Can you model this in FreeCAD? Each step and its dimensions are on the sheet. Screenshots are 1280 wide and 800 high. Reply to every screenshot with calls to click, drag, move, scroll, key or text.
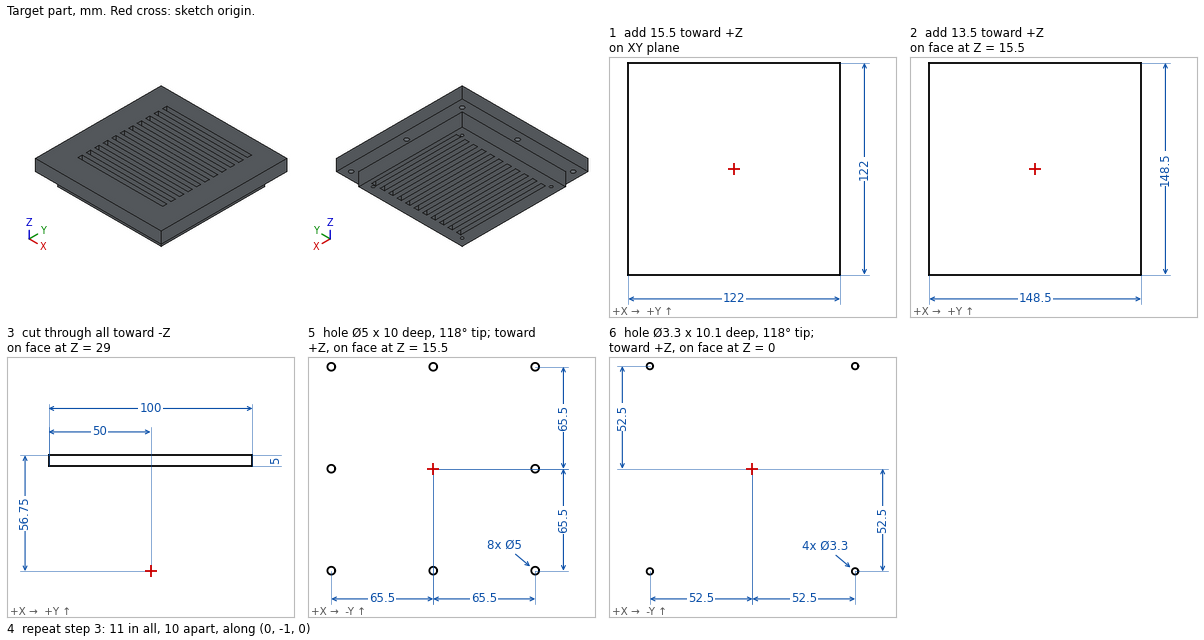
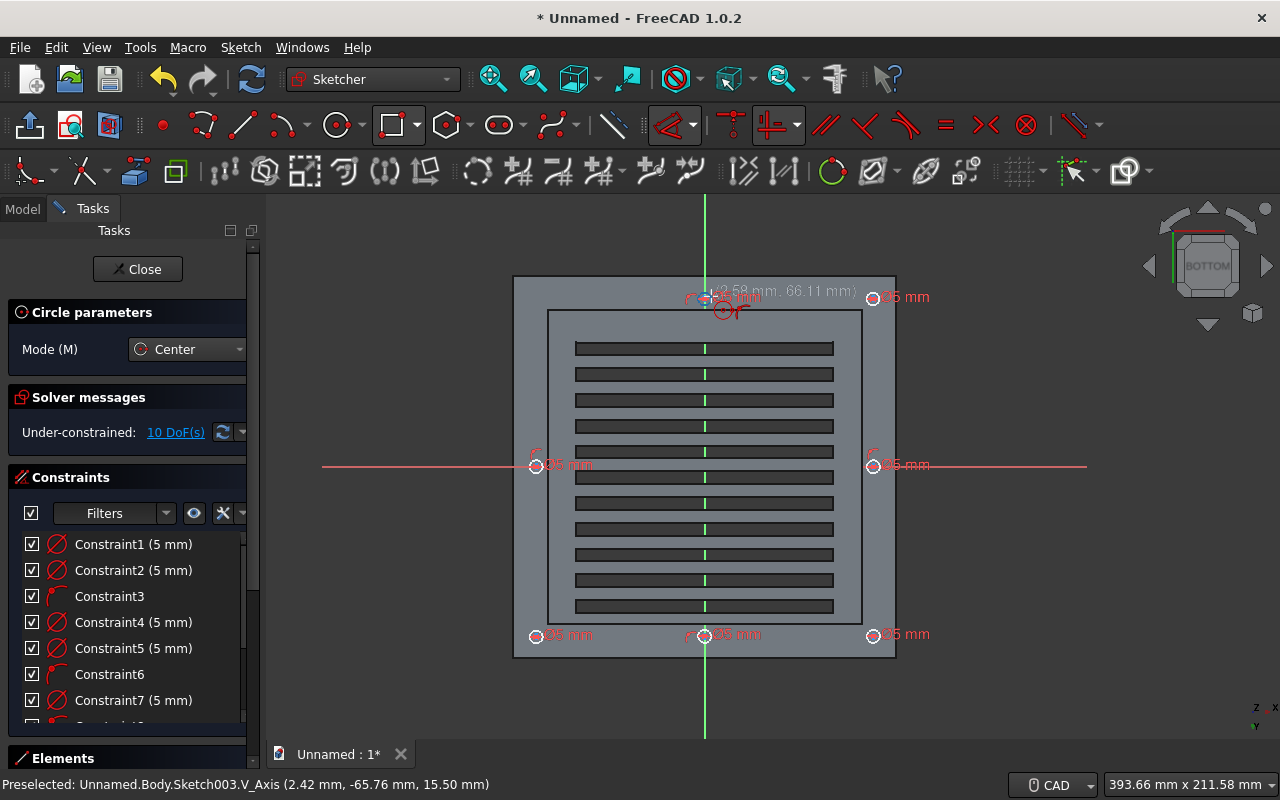
scroll(536, 298, up, 7)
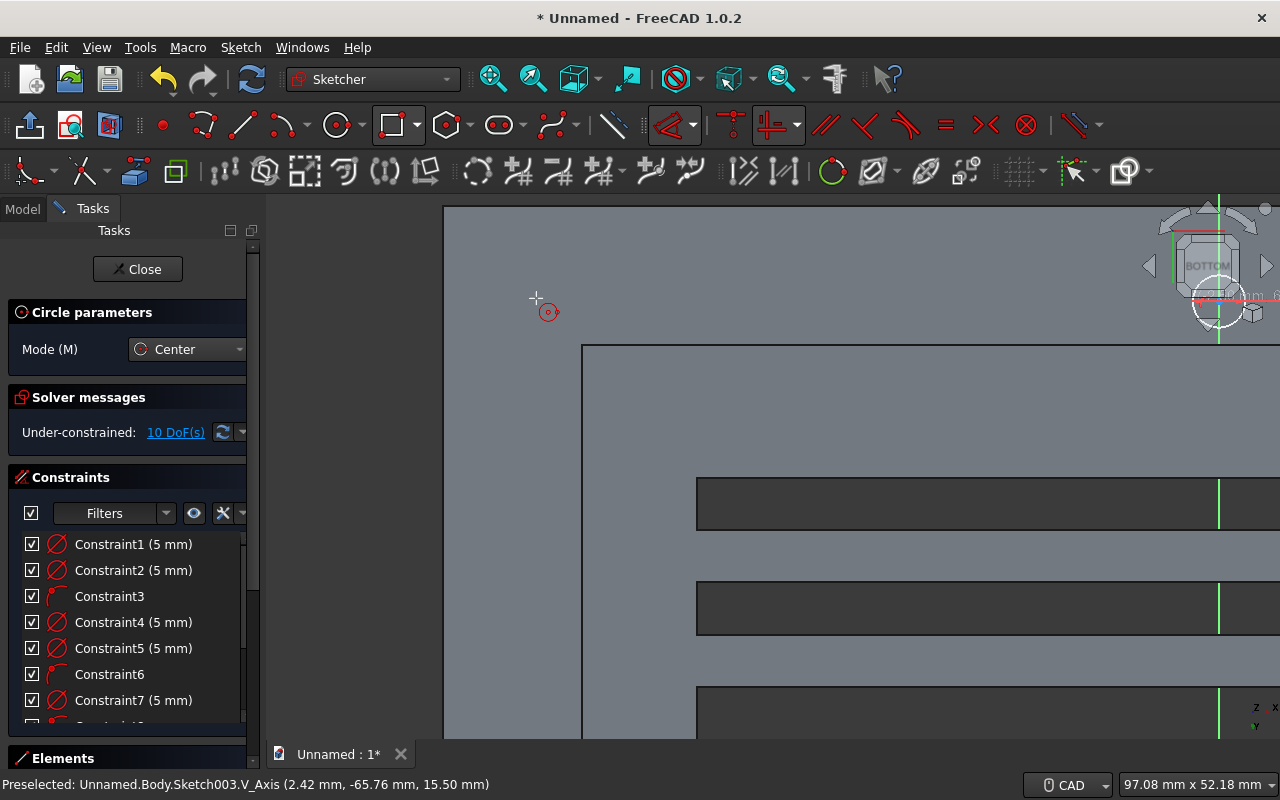
scroll(536, 298, down, 7)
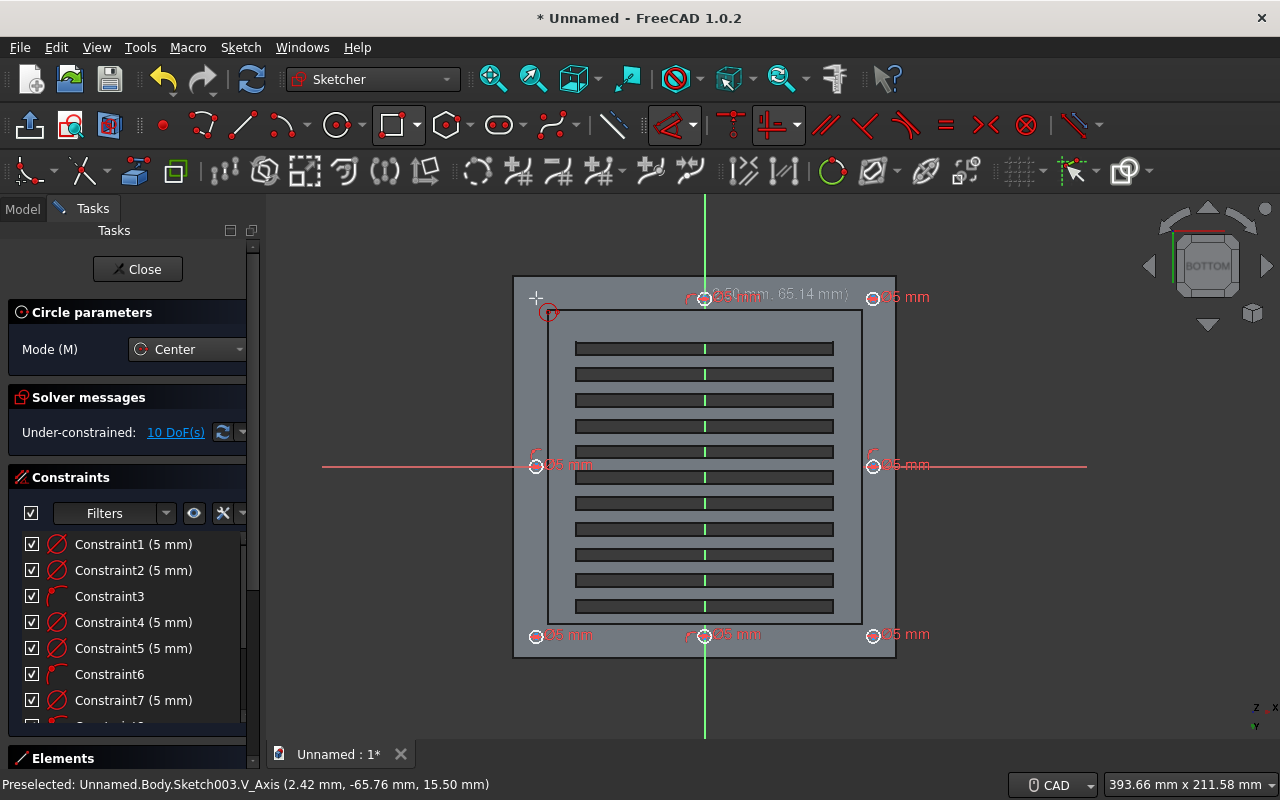
click(536, 298)
move(540, 294)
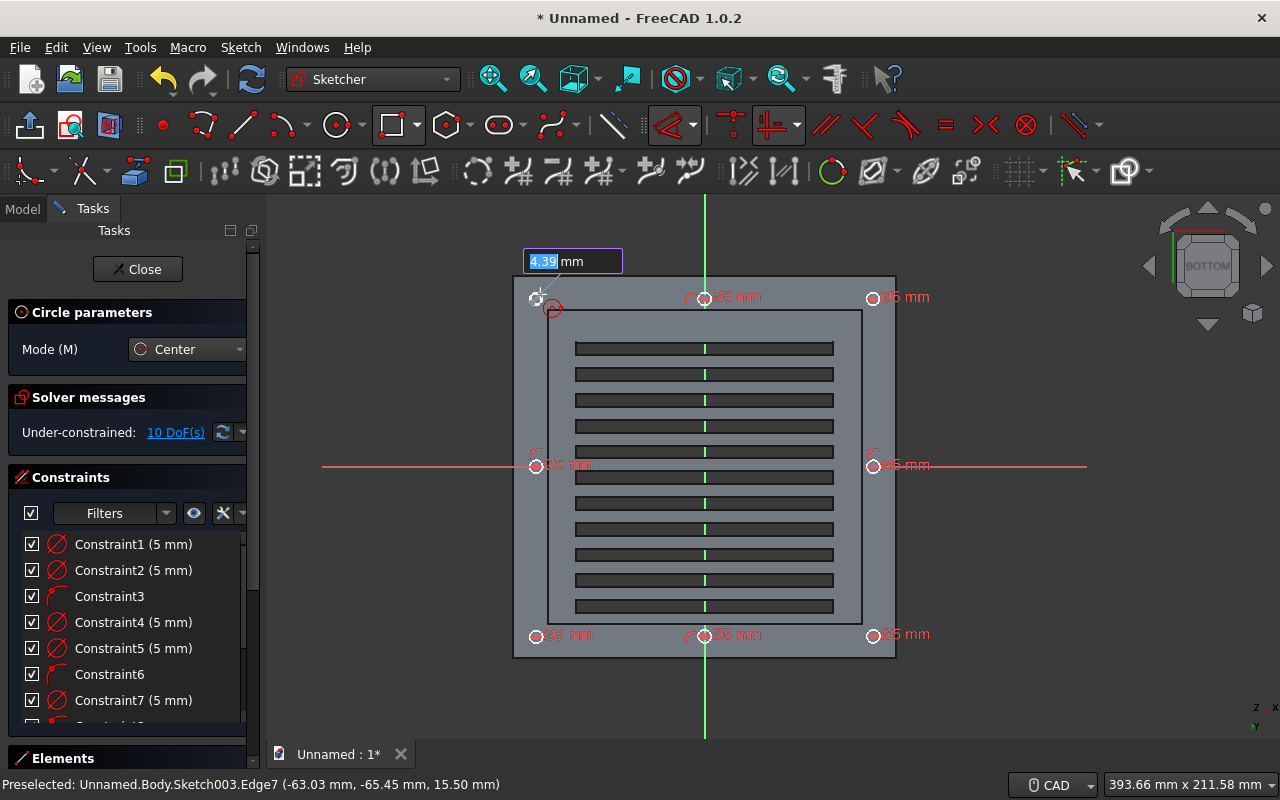
text(5)
key(Return)
key(Escape)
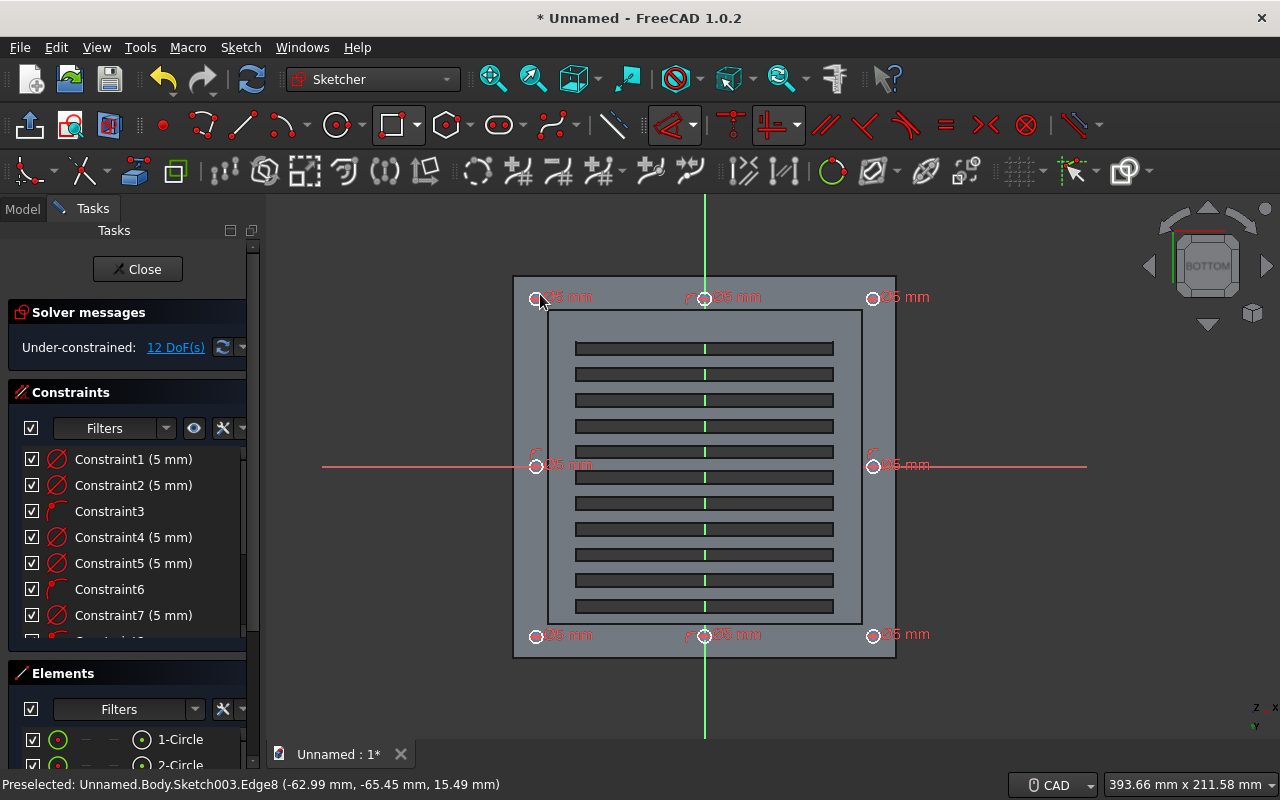
click(873, 636)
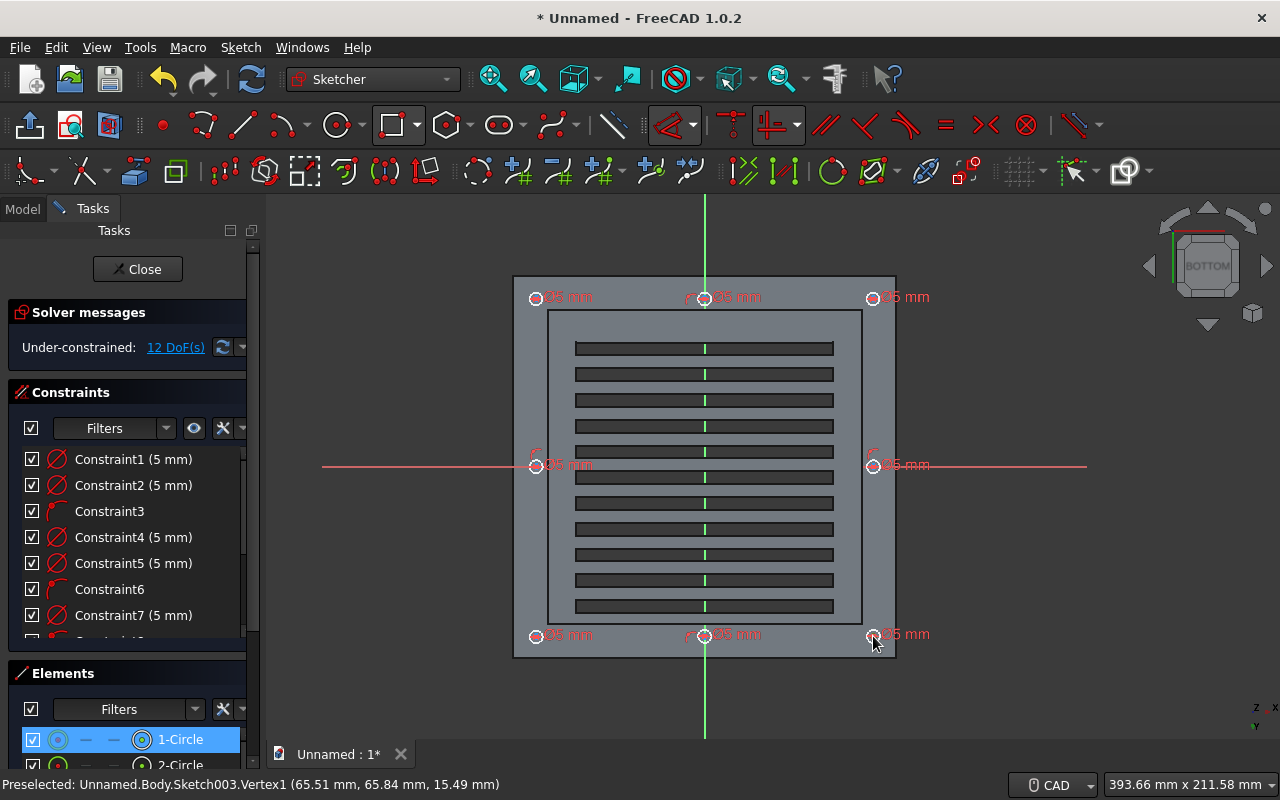
click(705, 636)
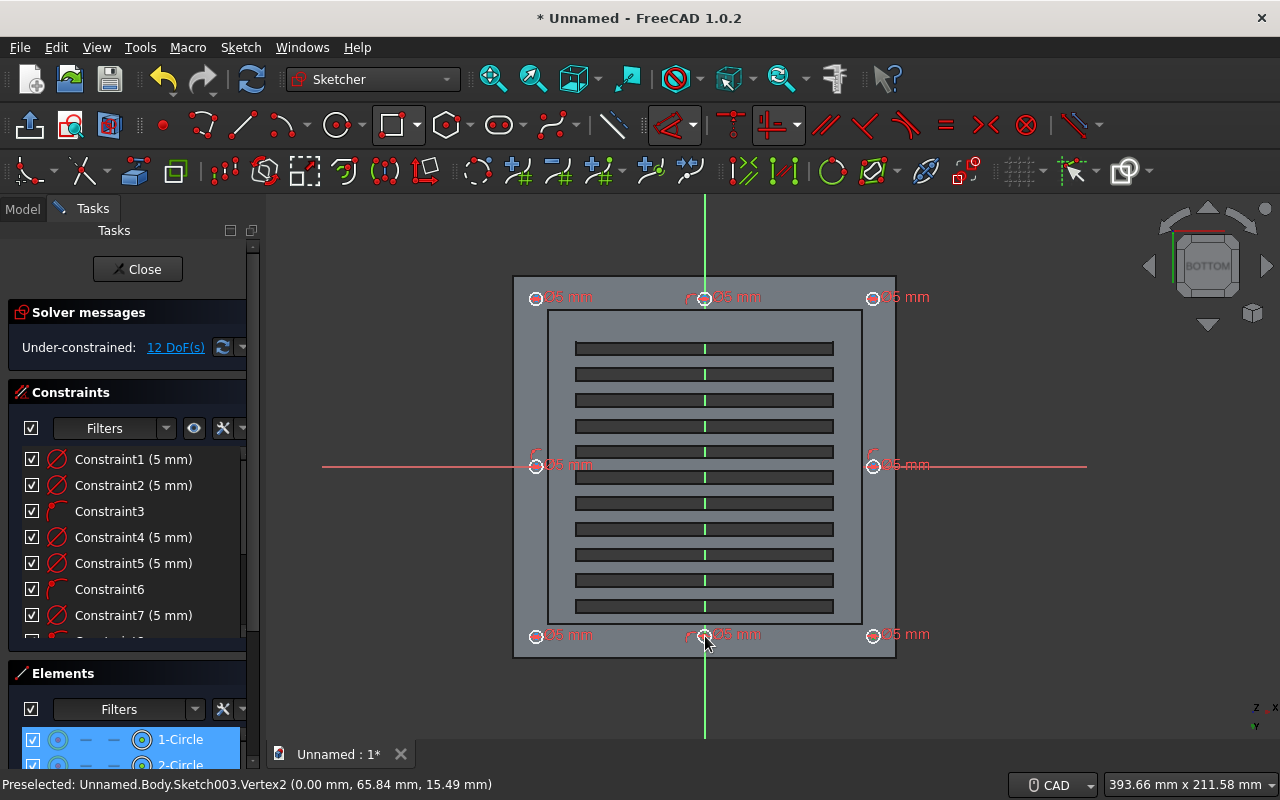
click(800, 126)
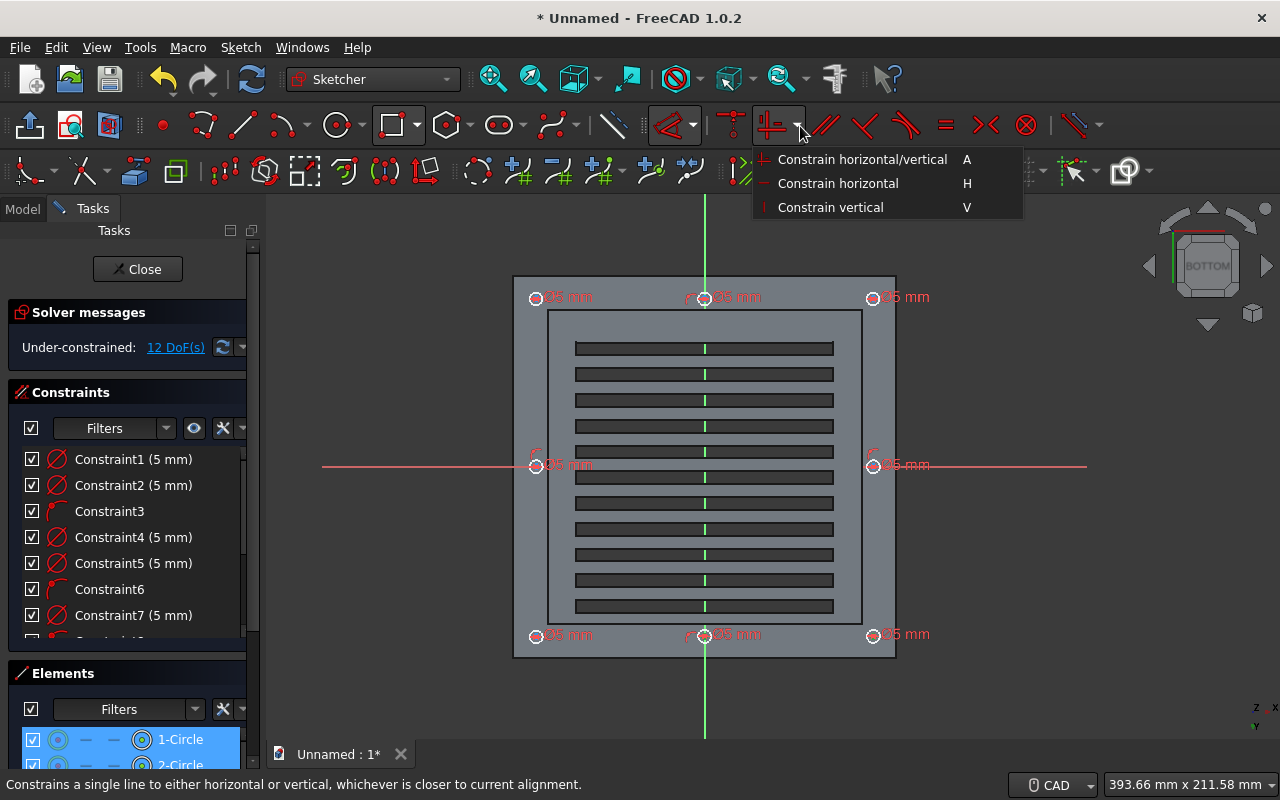
click(888, 183)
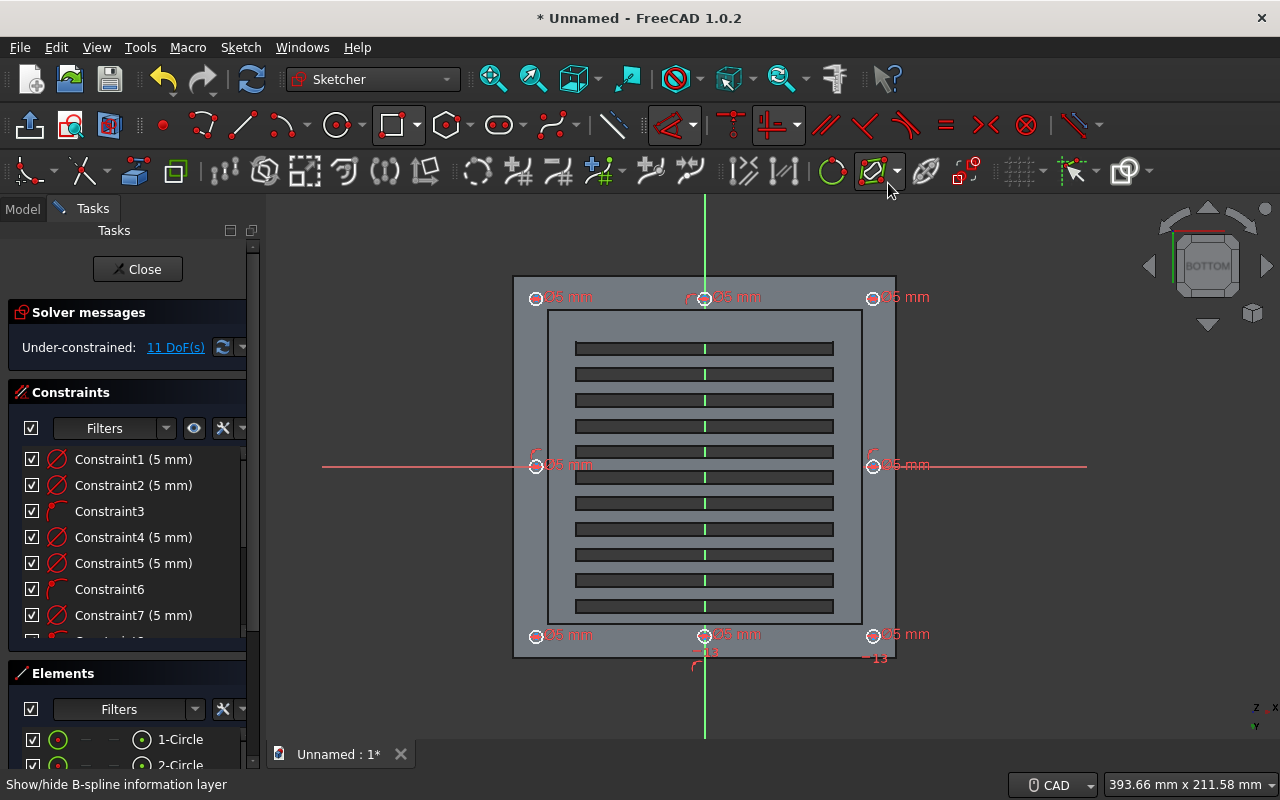
click(705, 636)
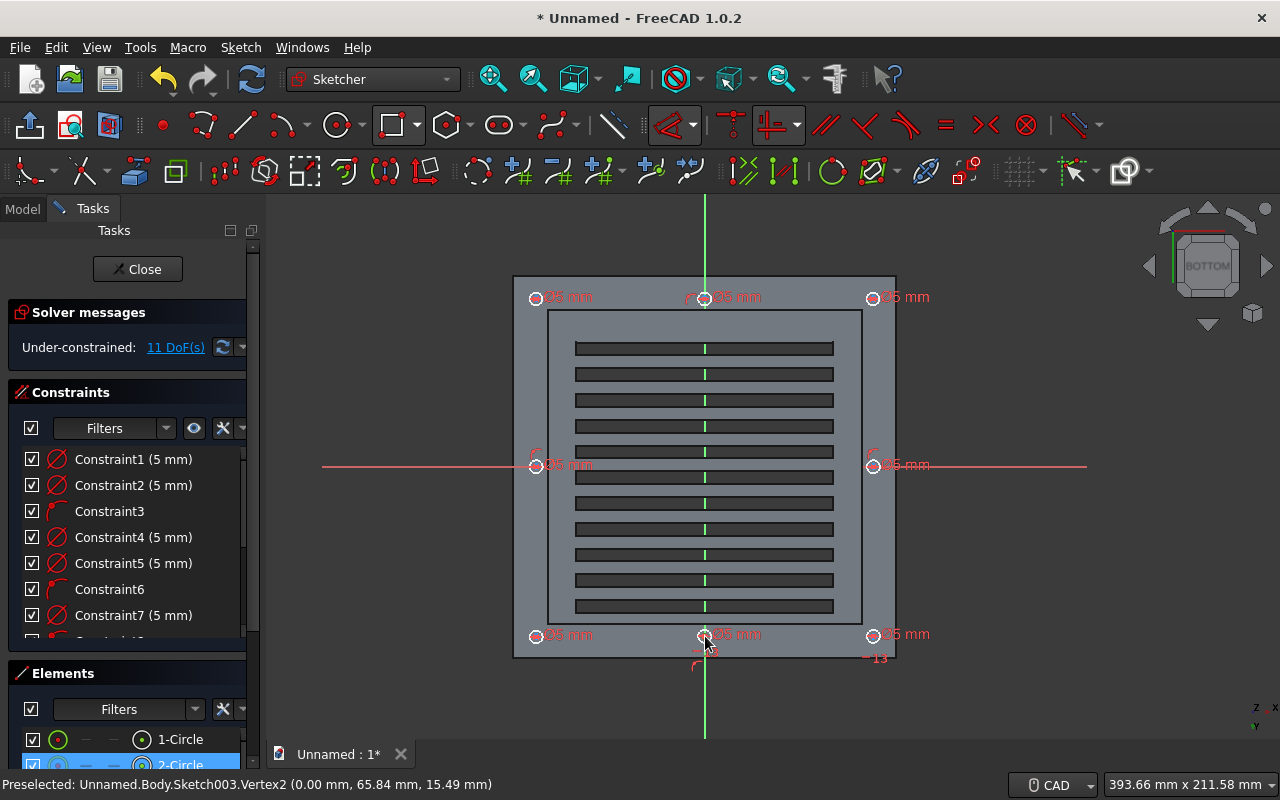
click(536, 637)